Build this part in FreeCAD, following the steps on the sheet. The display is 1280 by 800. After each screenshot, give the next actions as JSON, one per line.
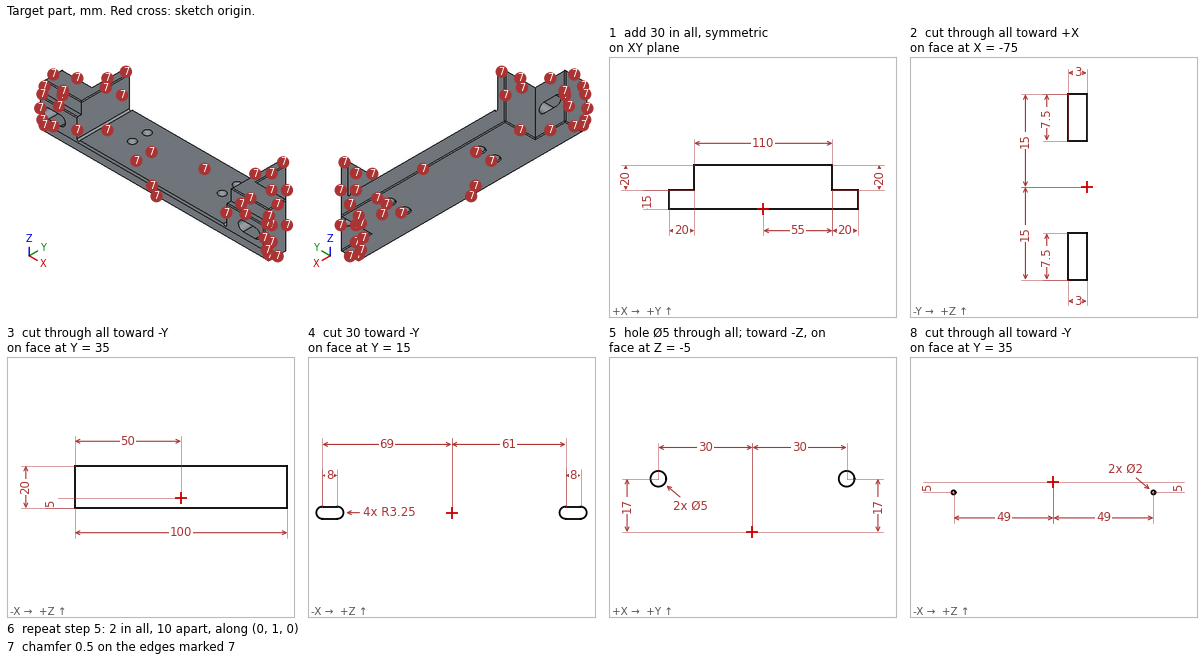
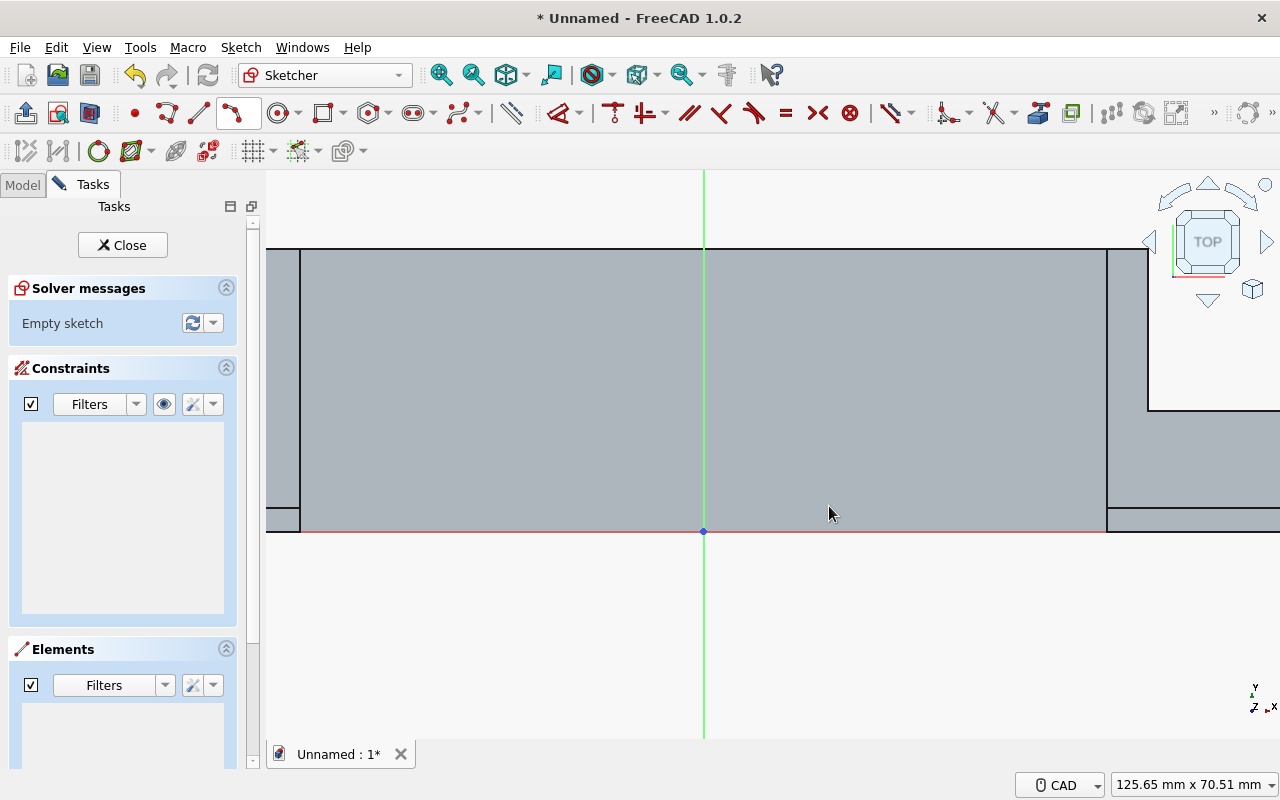
{"action": "key", "text": "g c"}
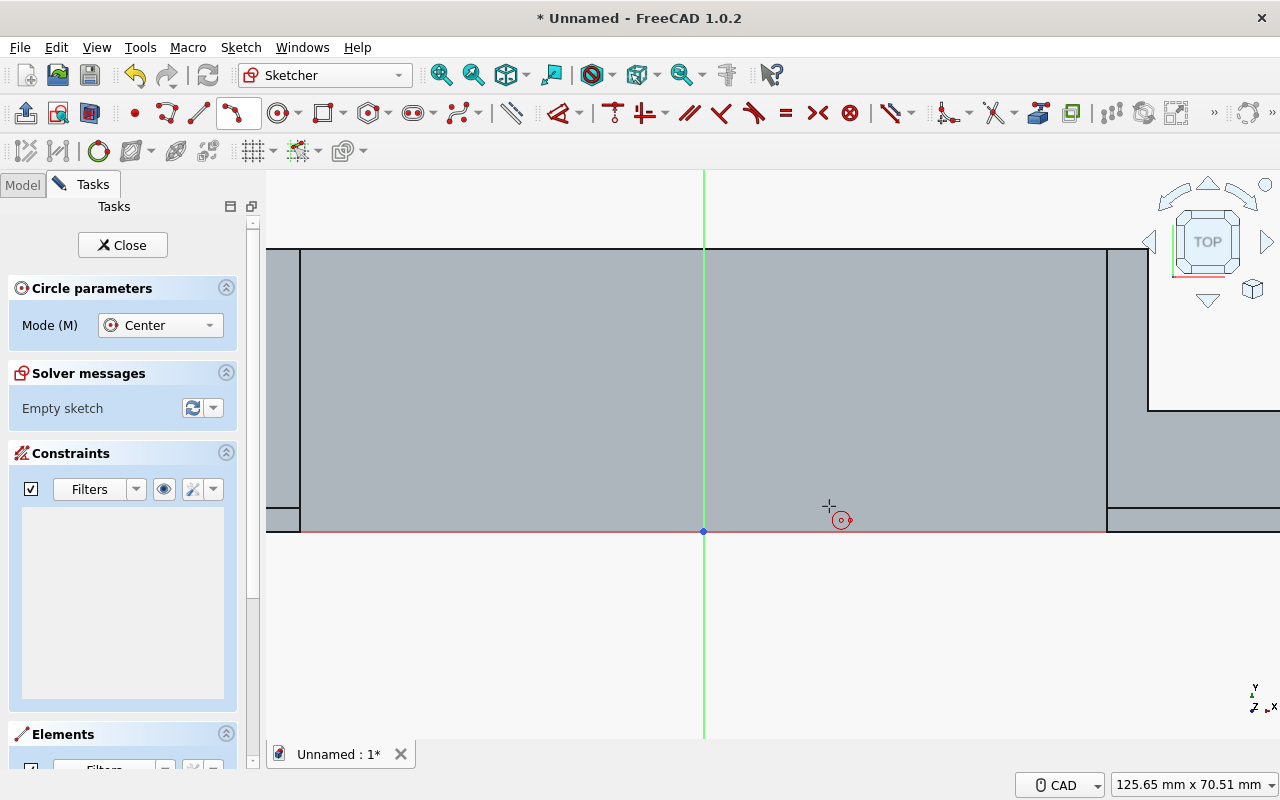
{"action": "left_click", "coordinate": [462, 395]}
{"action": "left_click", "coordinate": [476, 380]}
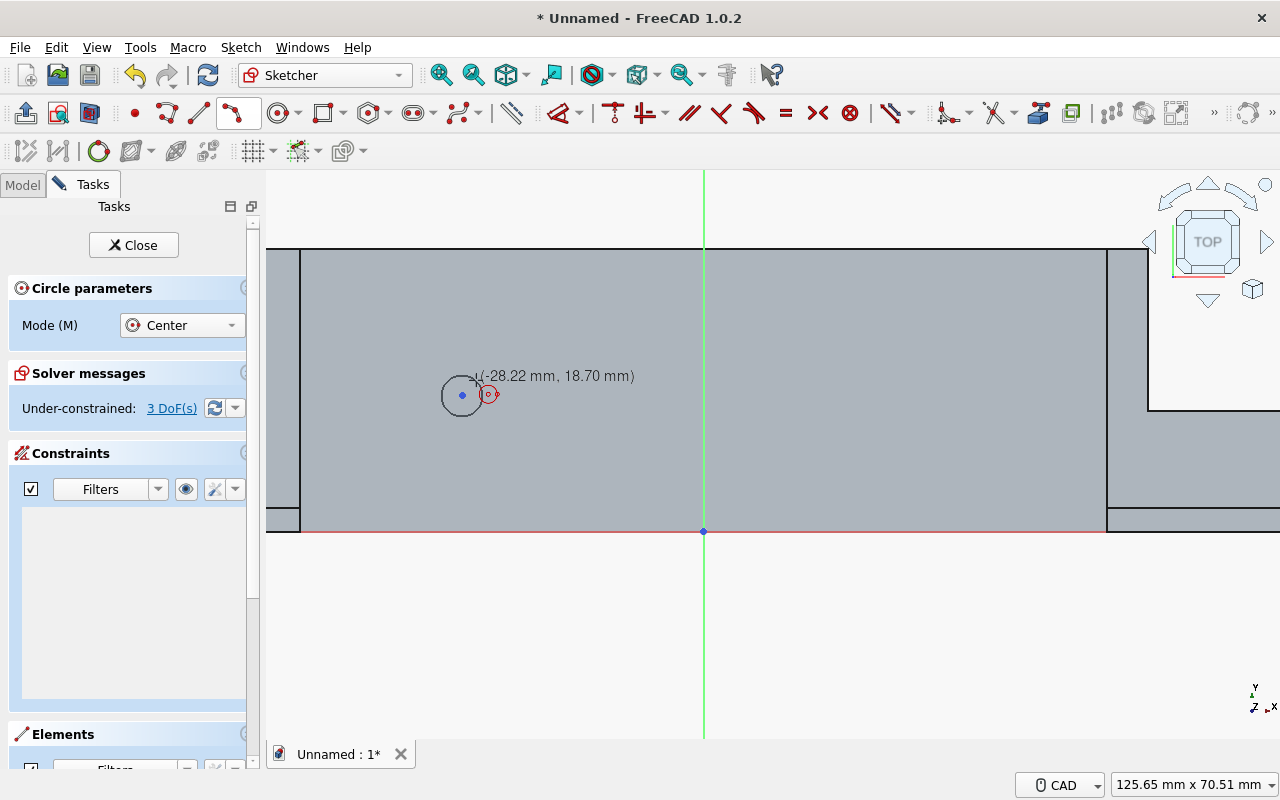
{"action": "left_click", "coordinate": [946, 395]}
{"action": "left_click", "coordinate": [960, 380]}
{"action": "key", "text": "Escape"}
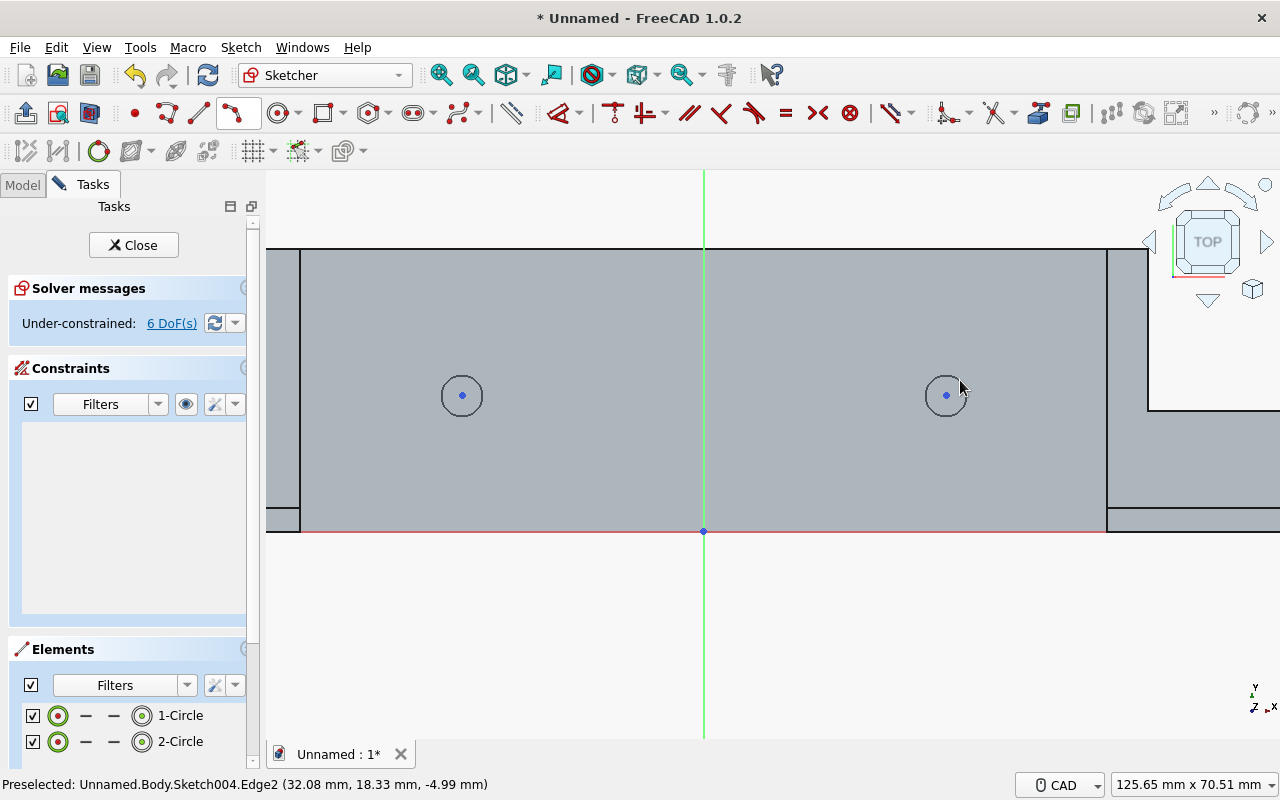
{"action": "left_click", "coordinate": [476, 381]}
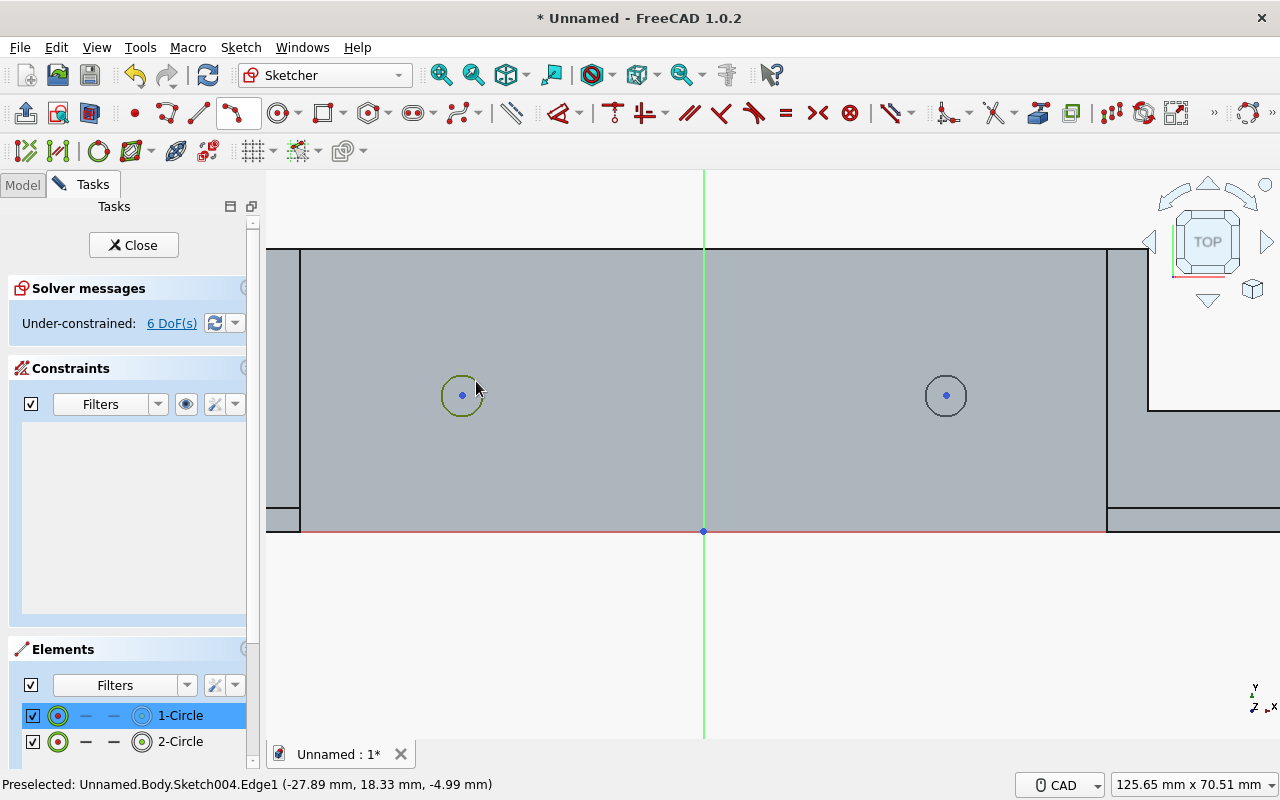
{"action": "left_click", "coordinate": [960, 381]}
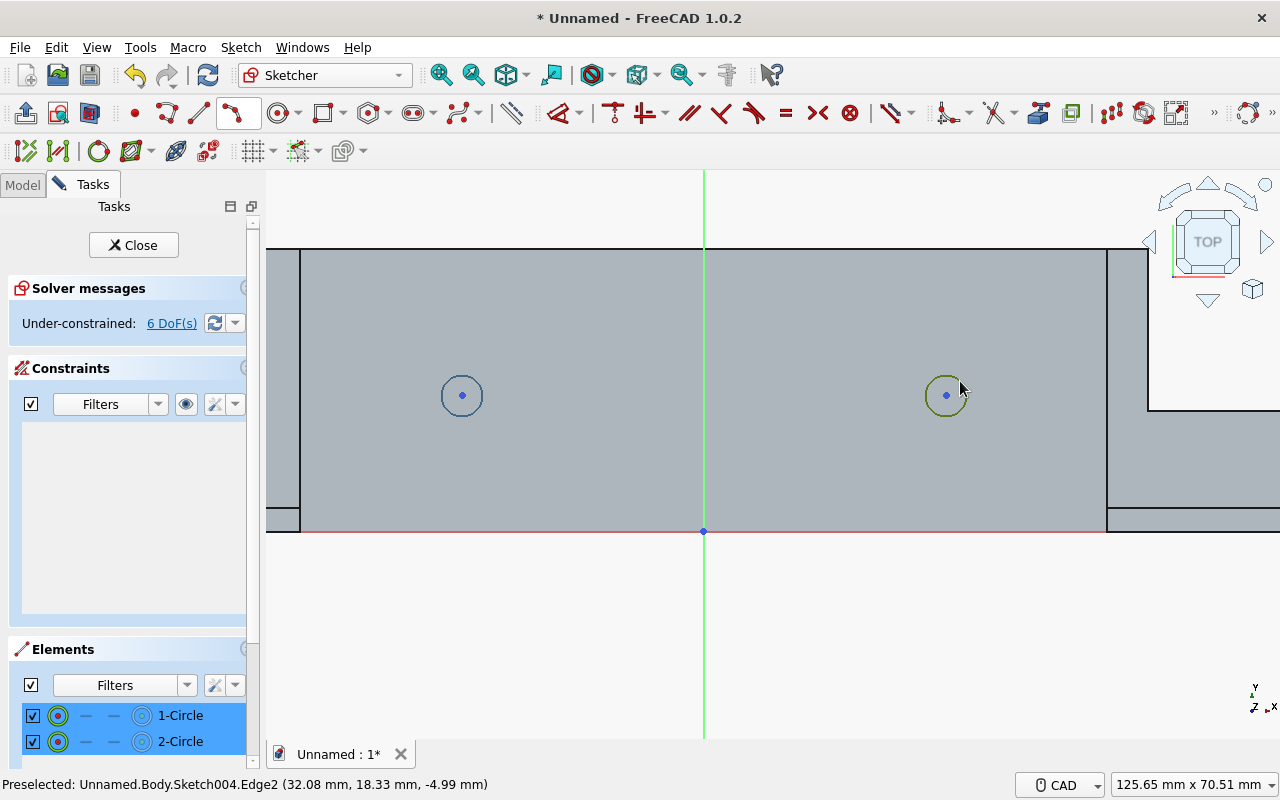
{"action": "left_click", "coordinate": [786, 114]}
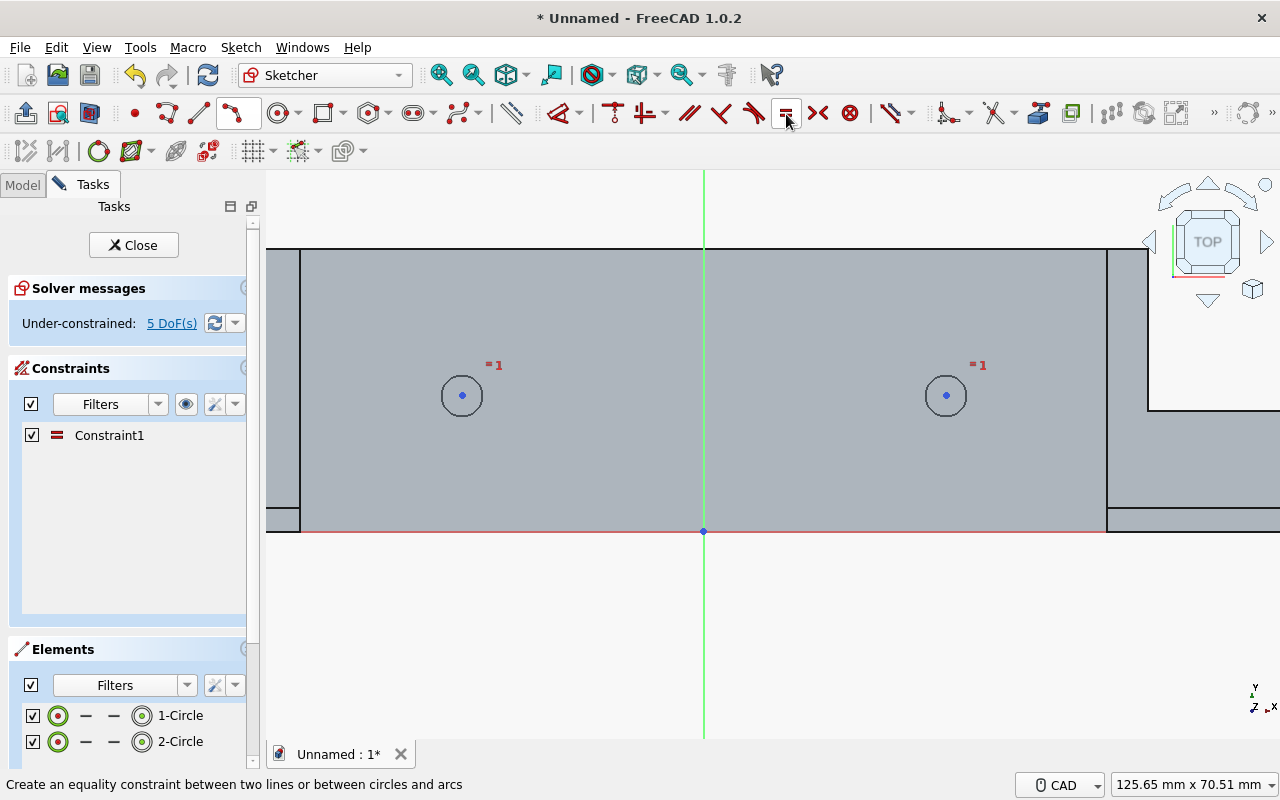
{"action": "key", "text": "d"}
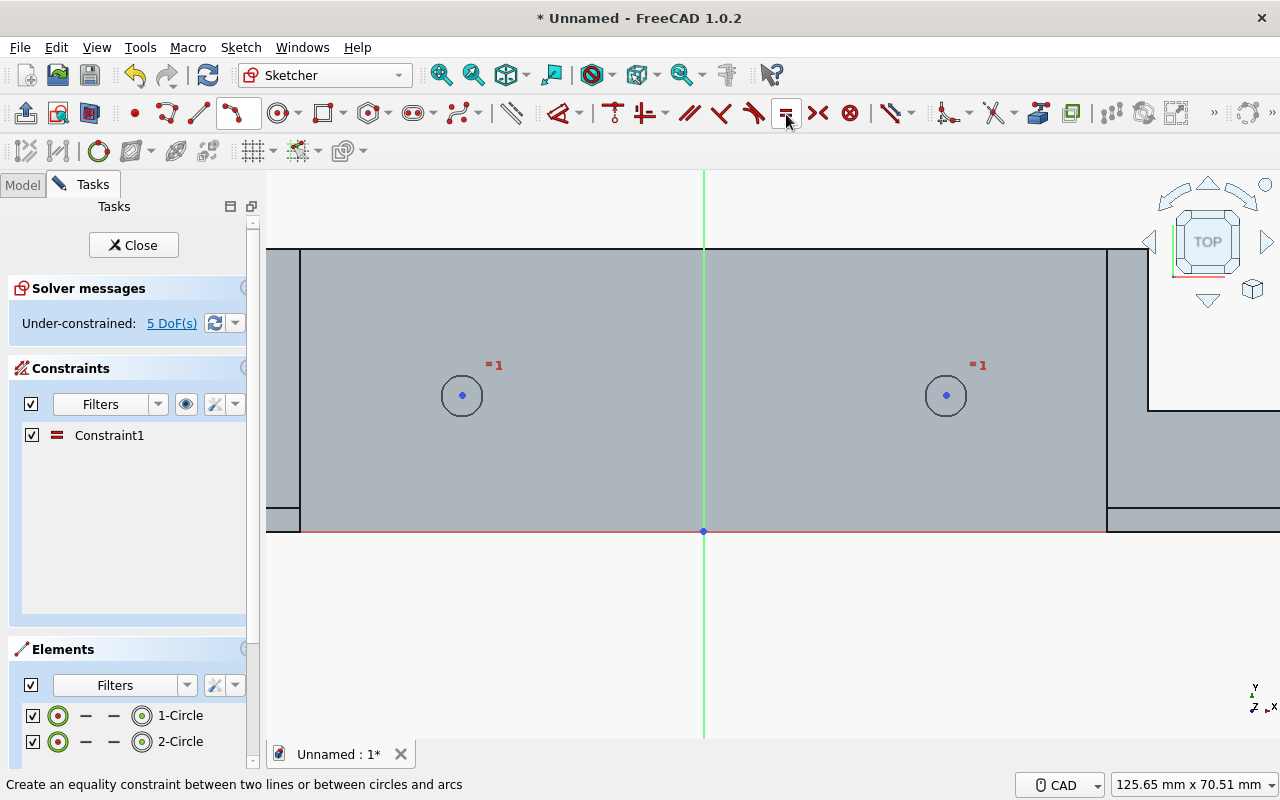
{"action": "left_click", "coordinate": [476, 381]}
{"action": "left_click", "coordinate": [498, 358]}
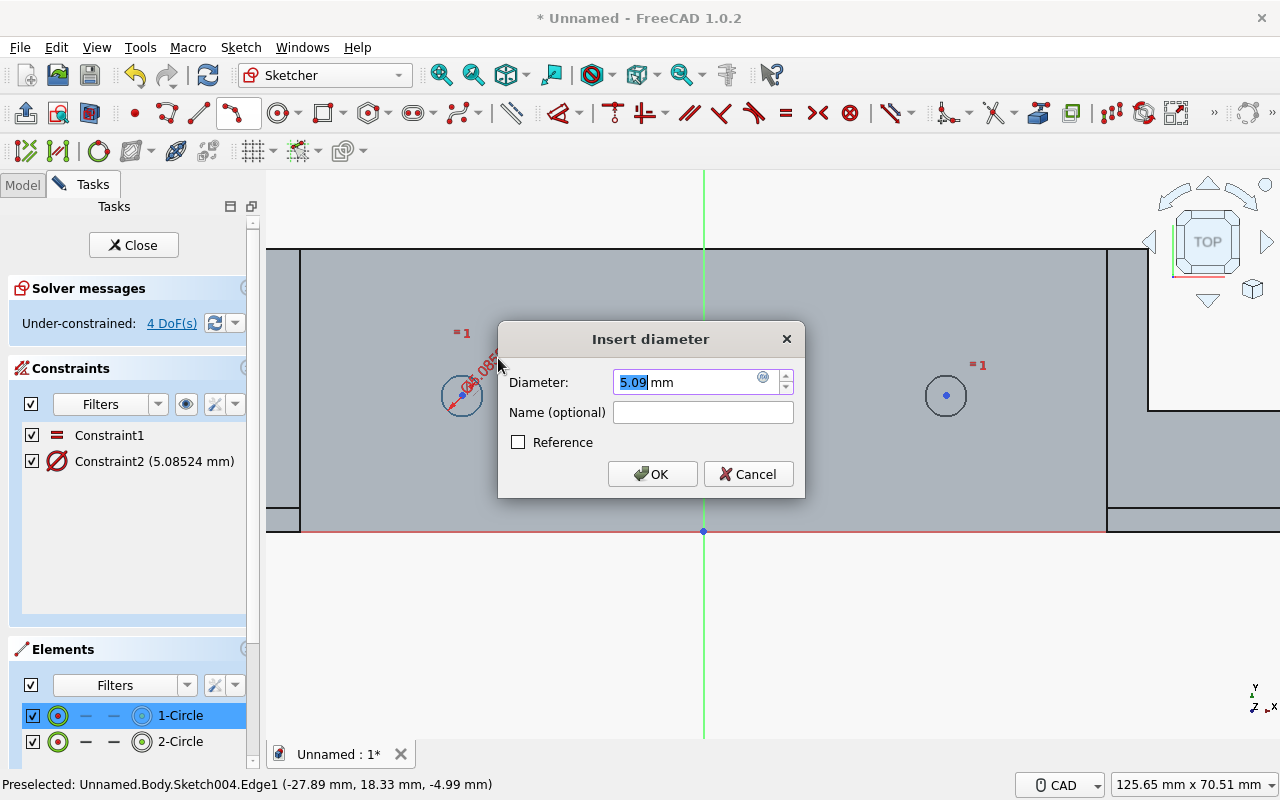
{"action": "type", "text": "5"}
{"action": "key", "text": "Return"}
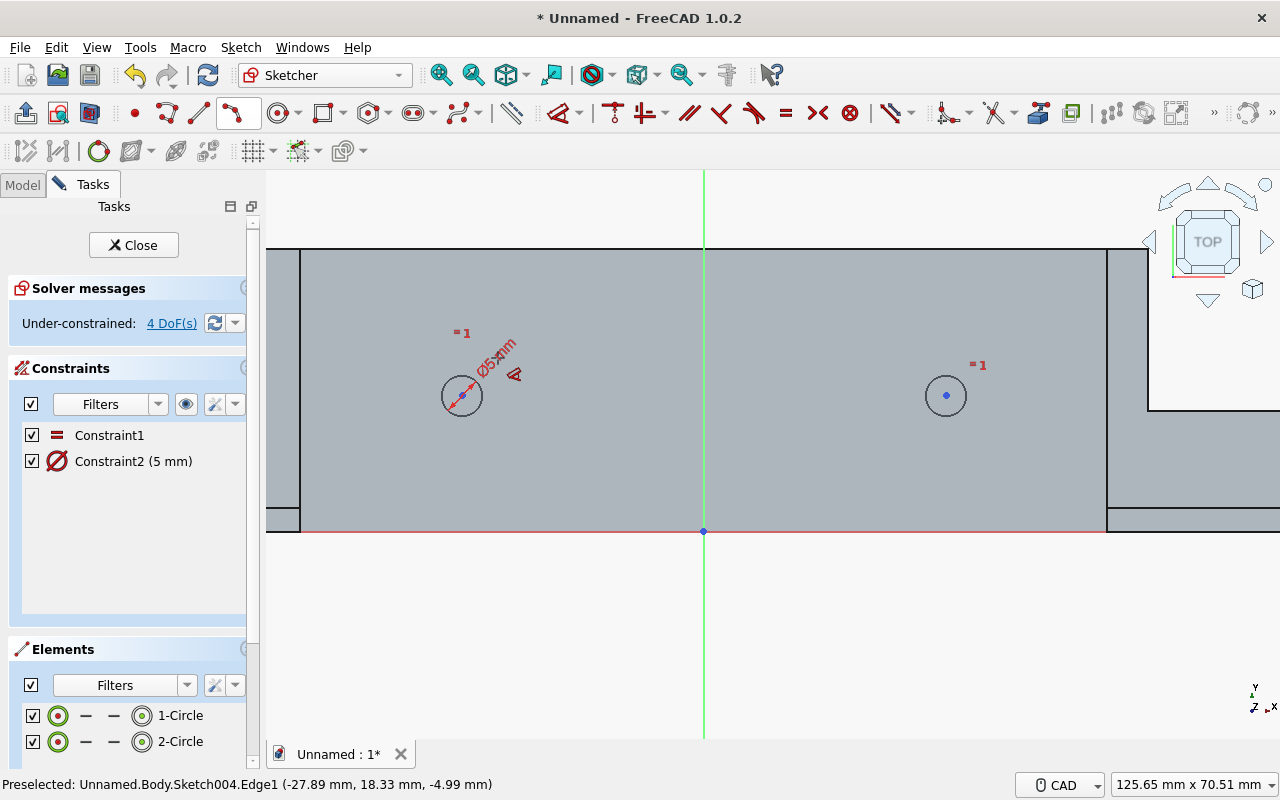
{"action": "left_click", "coordinate": [462, 396]}
{"action": "left_click", "coordinate": [583, 566]}